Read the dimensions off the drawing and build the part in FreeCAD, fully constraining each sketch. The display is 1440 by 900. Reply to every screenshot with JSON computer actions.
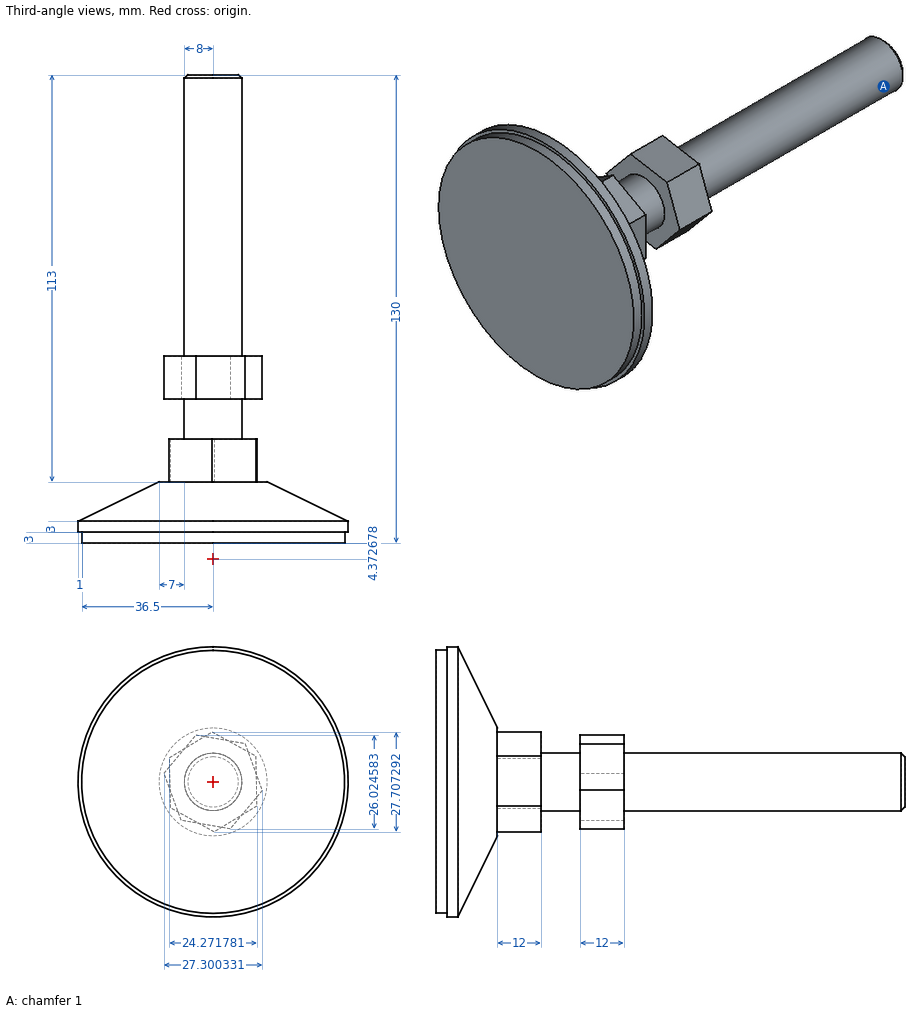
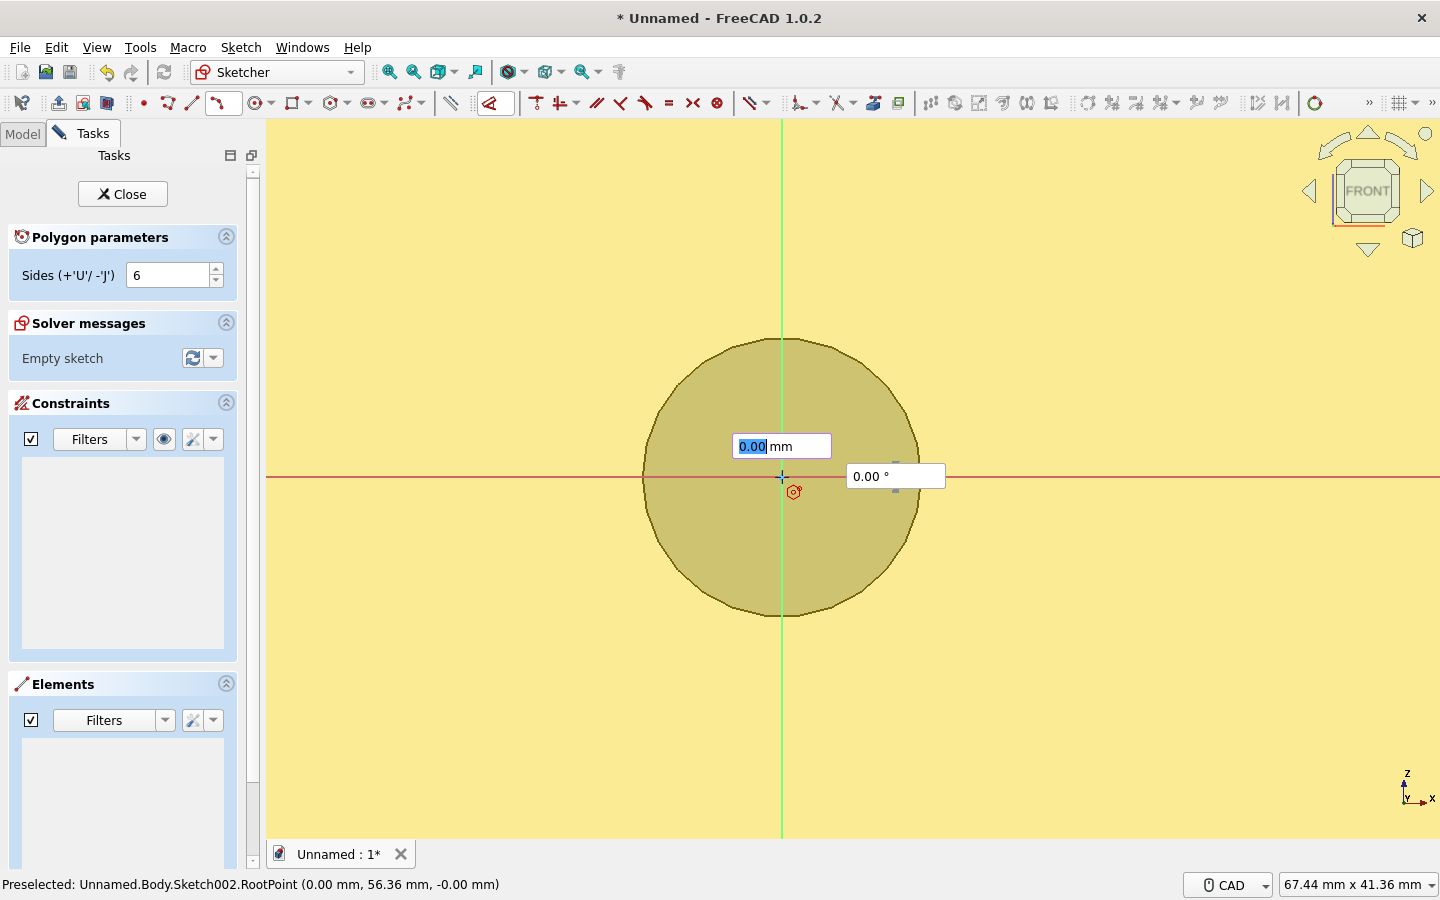
{"action": "left_click", "coordinate": [937, 292]}
{"action": "right_click", "coordinate": [937, 292]}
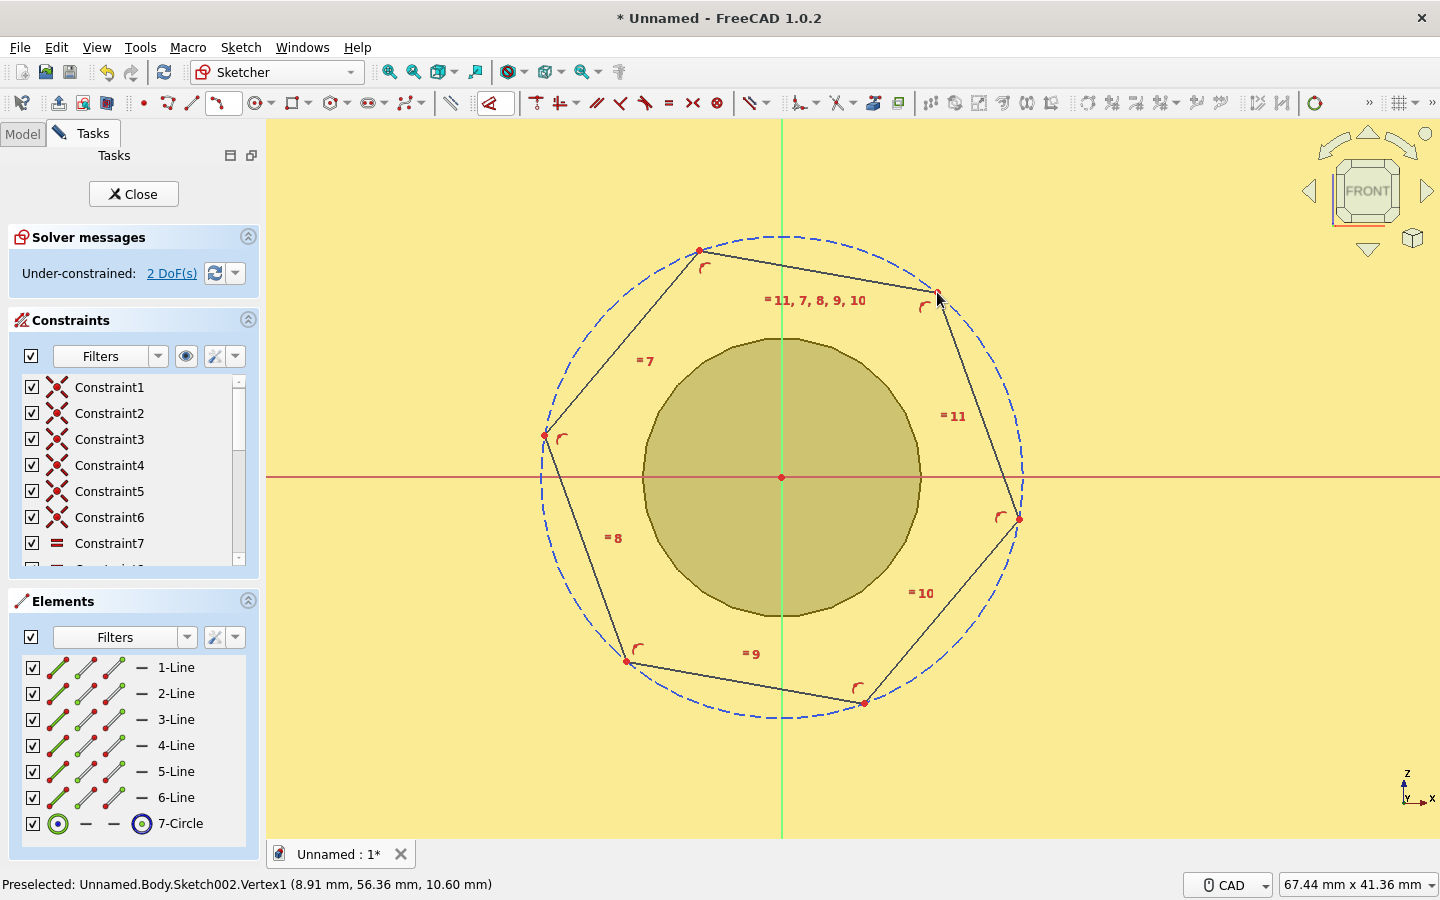
{"action": "left_click", "coordinate": [545, 435]}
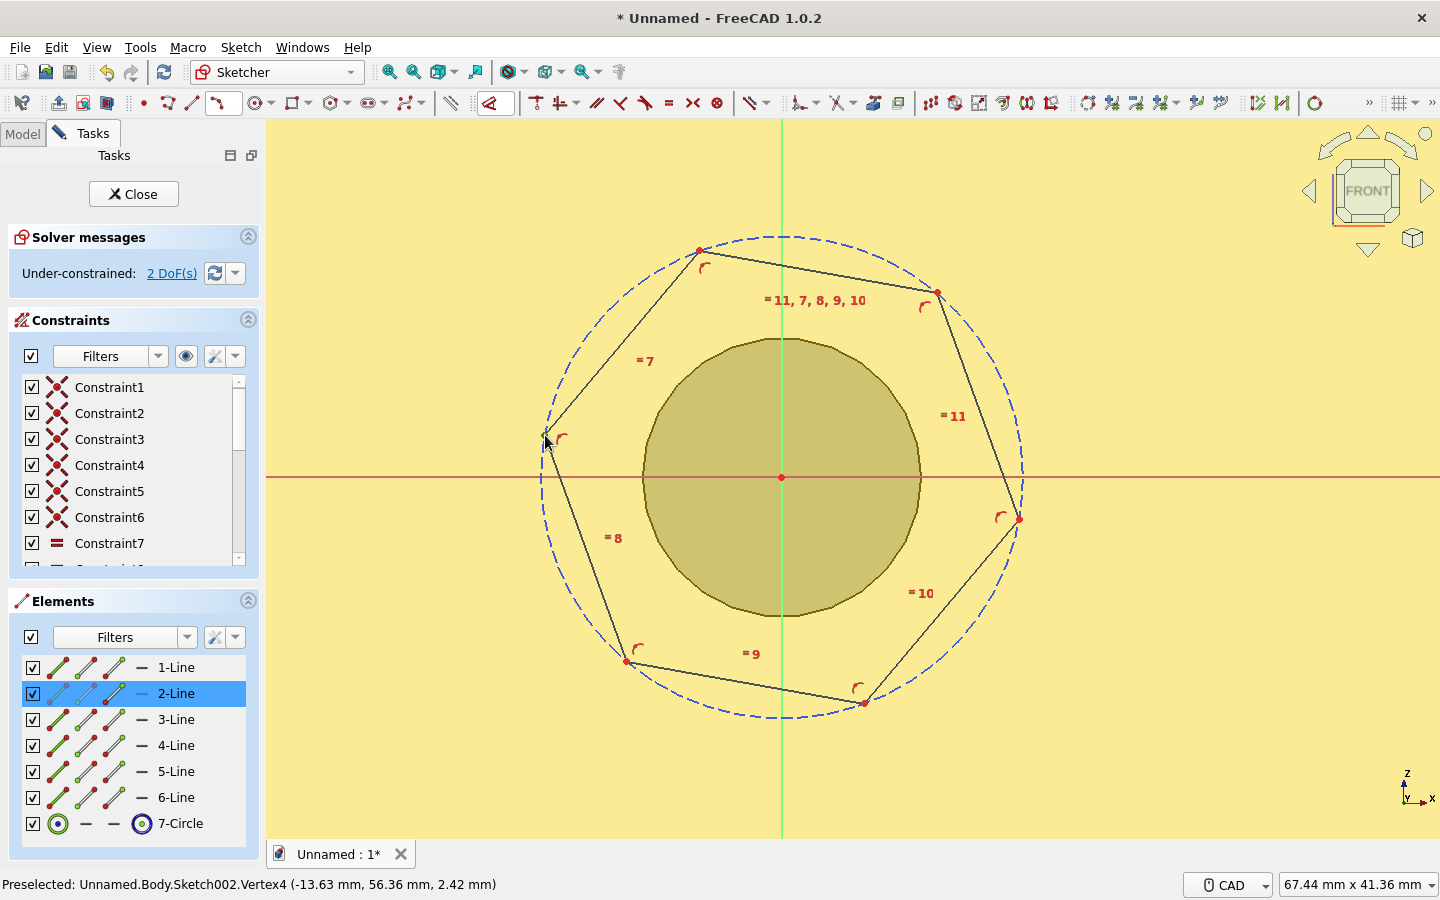
{"action": "left_click", "coordinate": [1019, 520]}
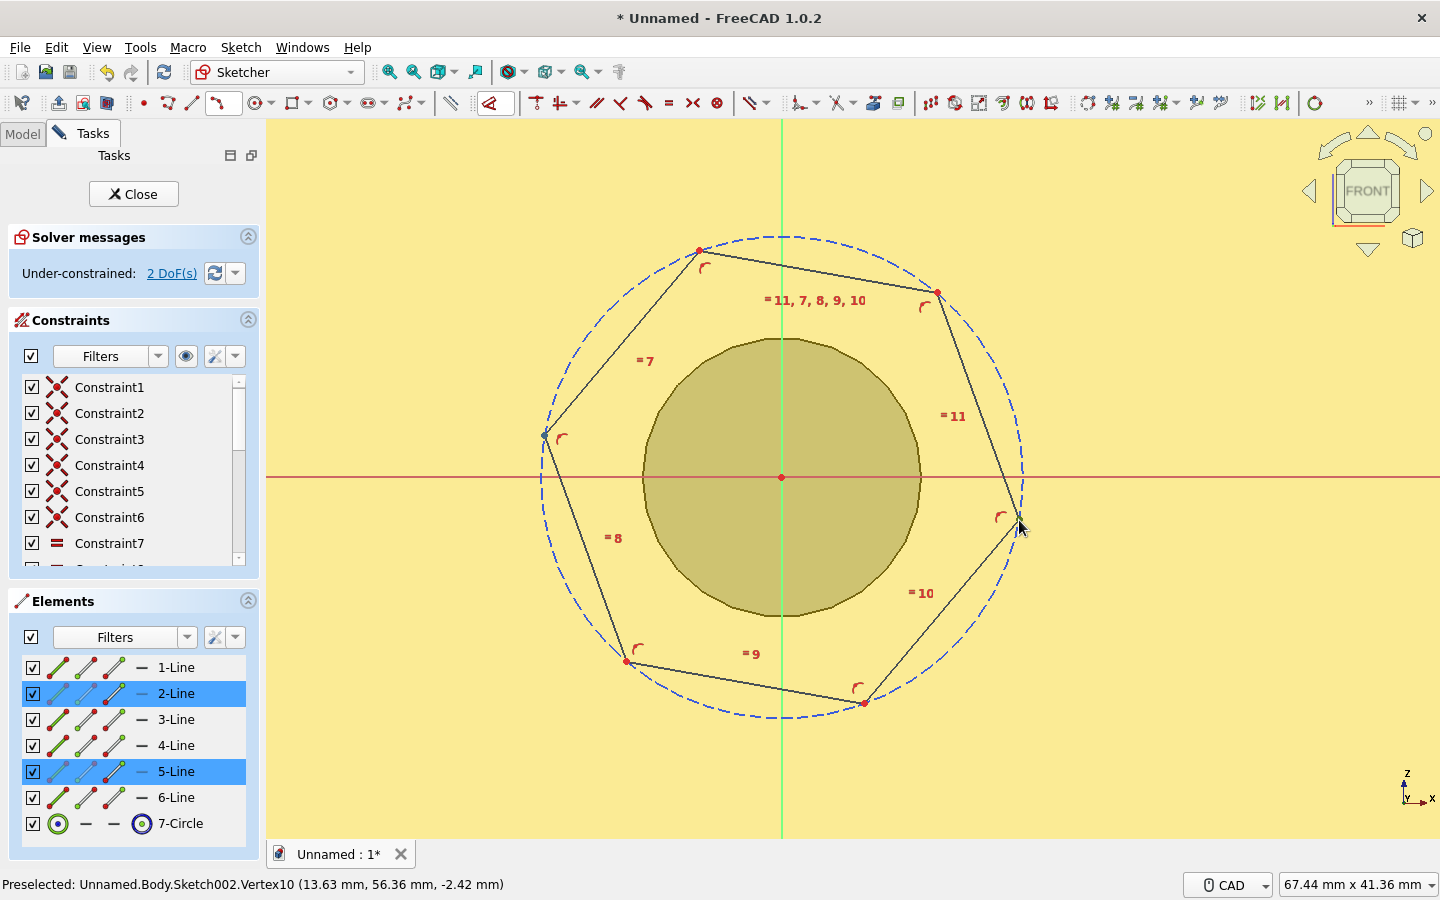
{"action": "left_click", "coordinate": [508, 104]}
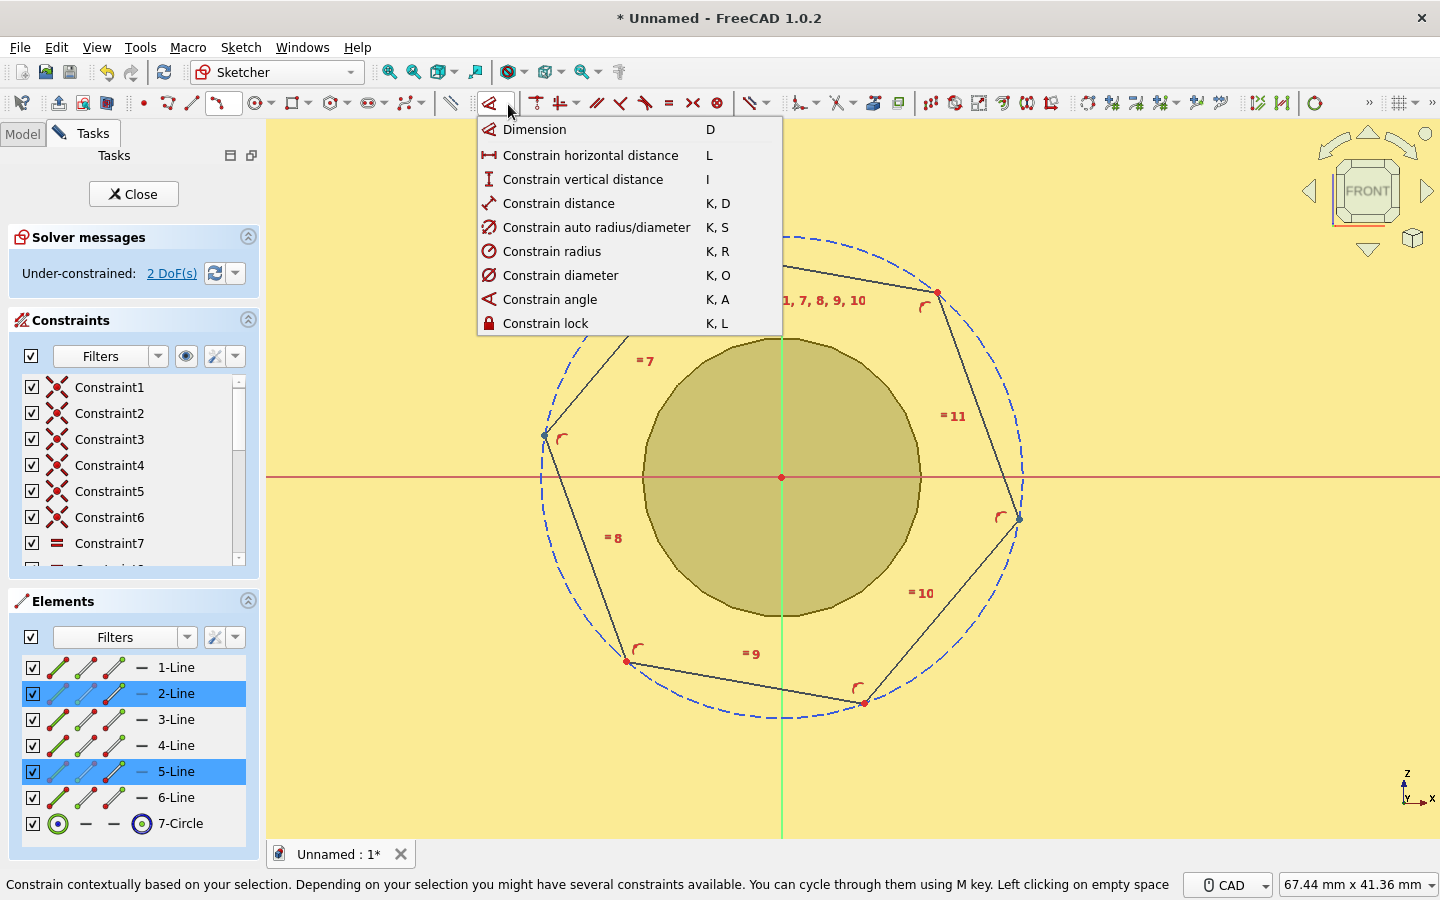
{"action": "left_click", "coordinate": [630, 155]}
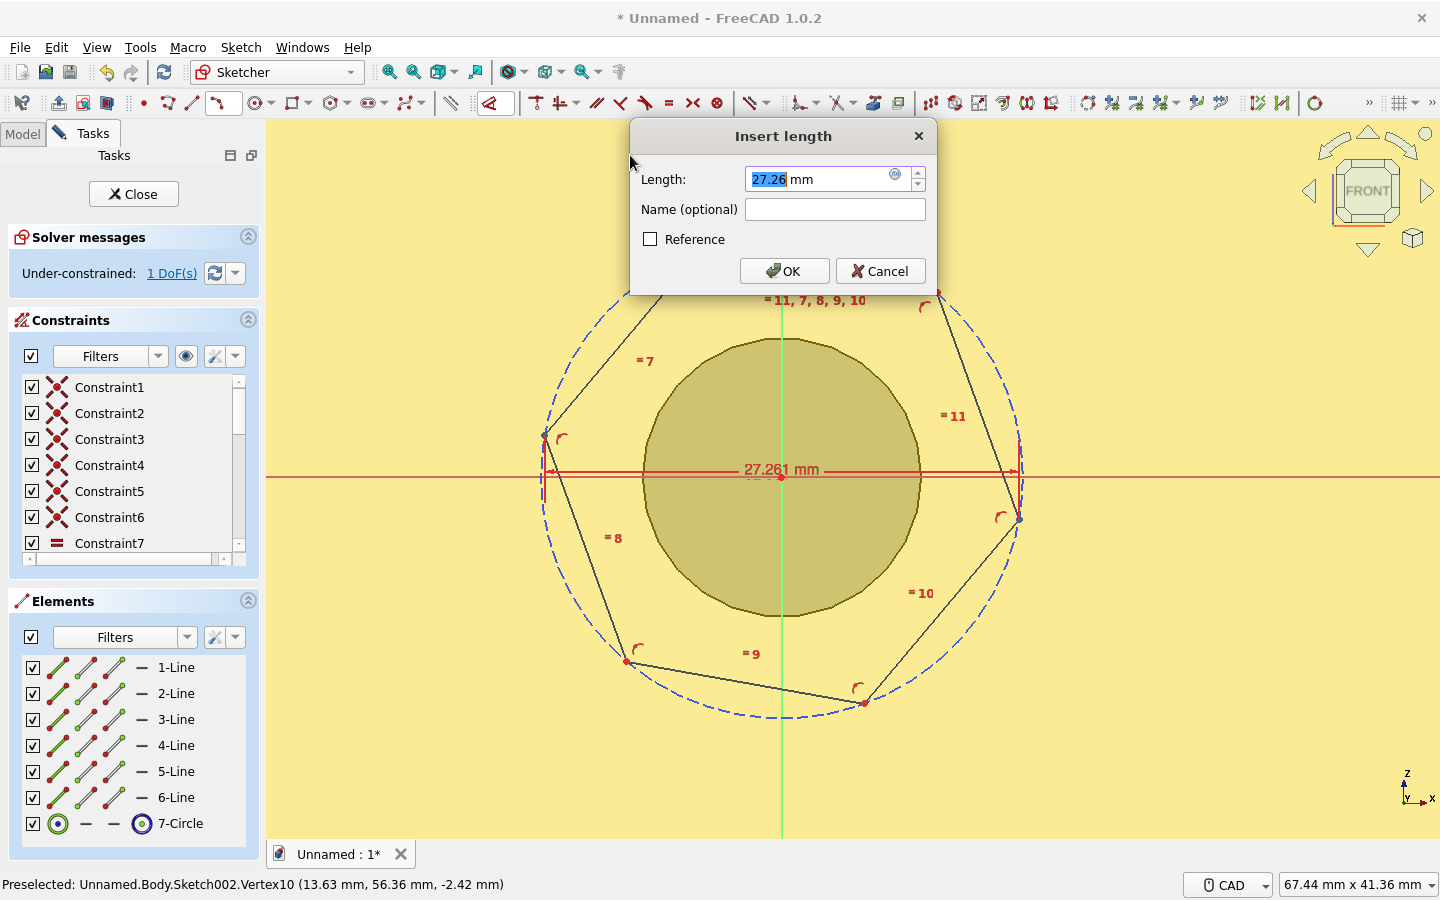
{"action": "type", "text": "27.300331"}
{"action": "key", "text": "Return"}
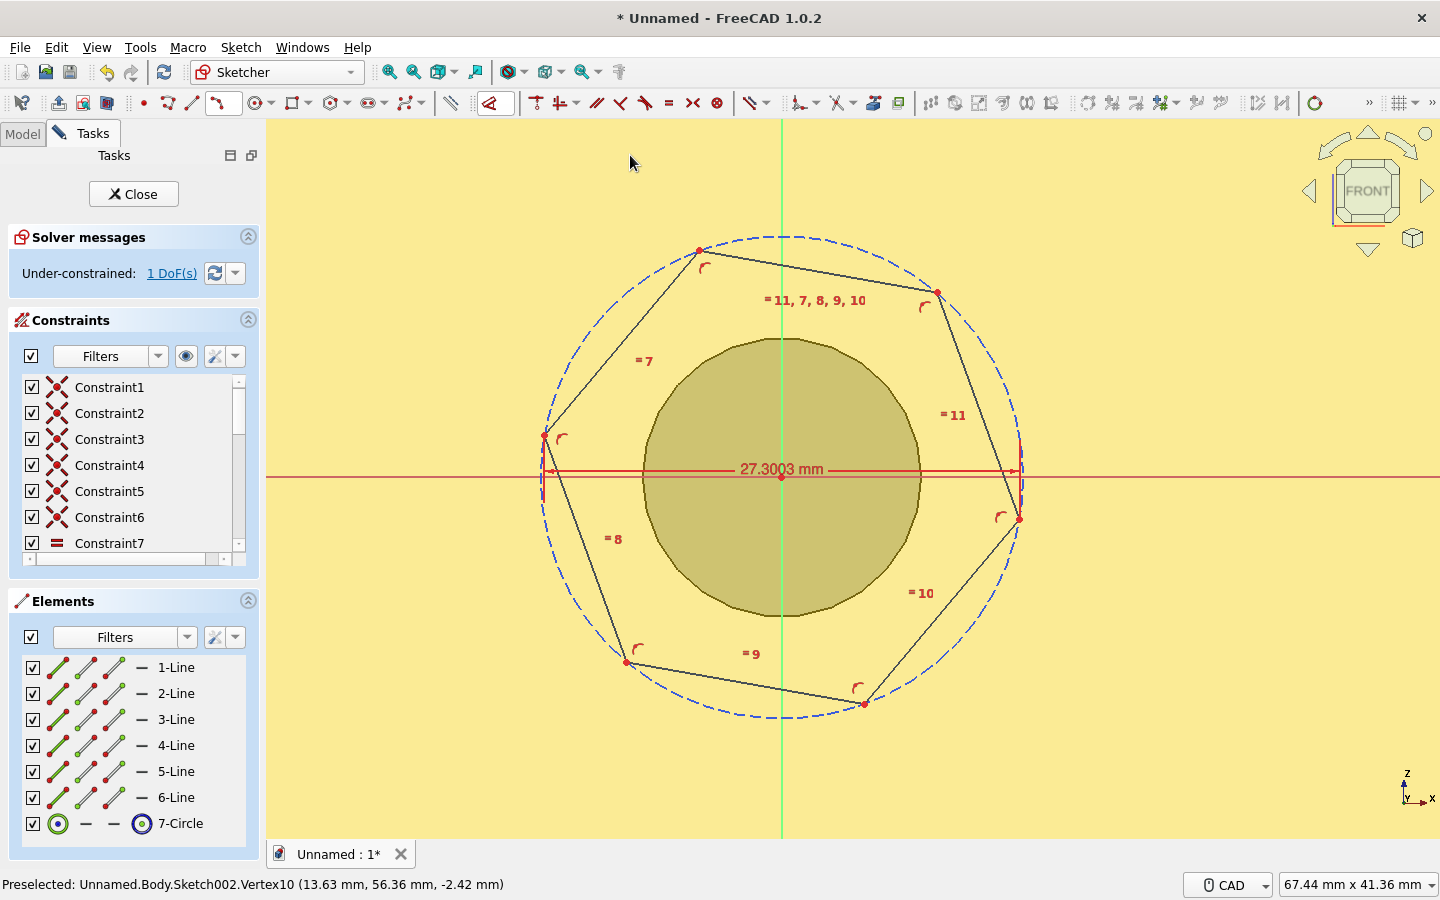
{"action": "left_click", "coordinate": [865, 704]}